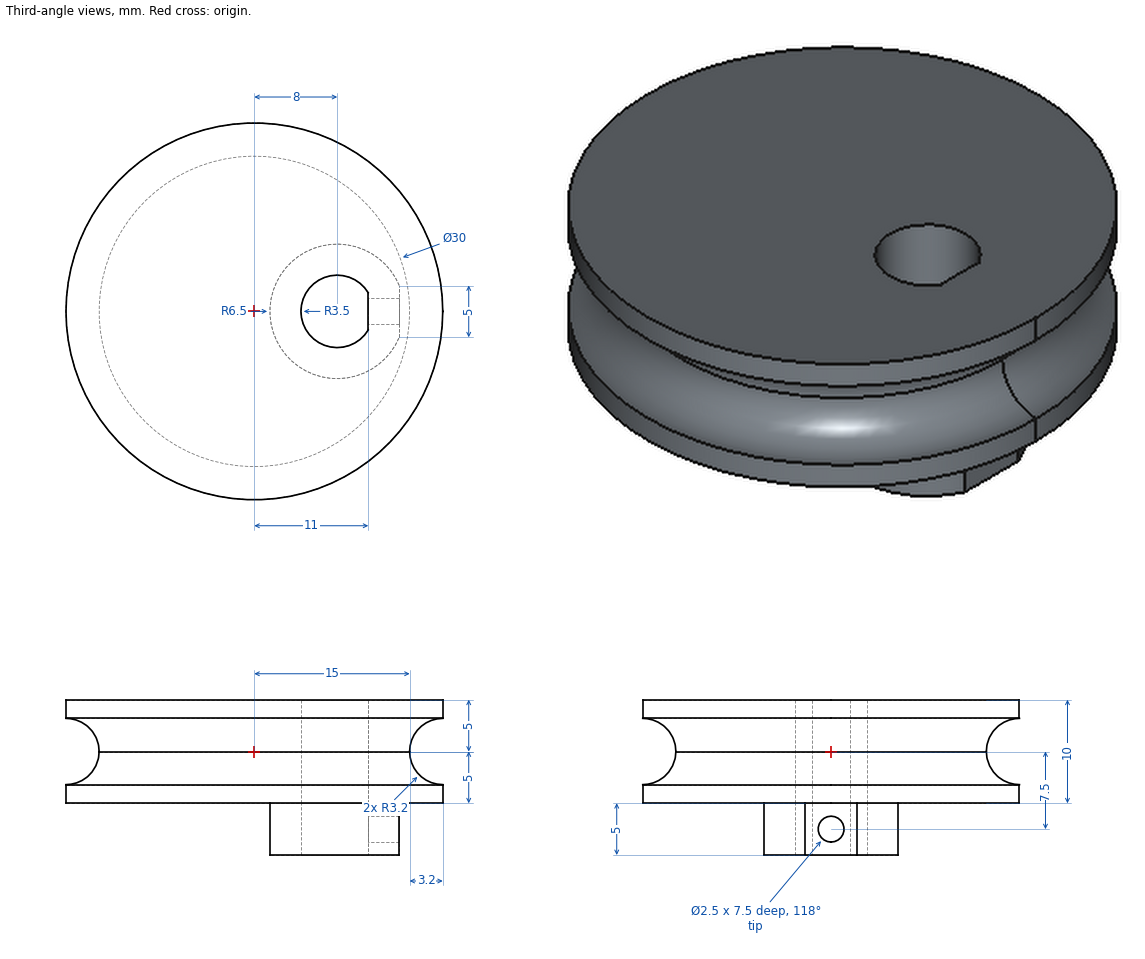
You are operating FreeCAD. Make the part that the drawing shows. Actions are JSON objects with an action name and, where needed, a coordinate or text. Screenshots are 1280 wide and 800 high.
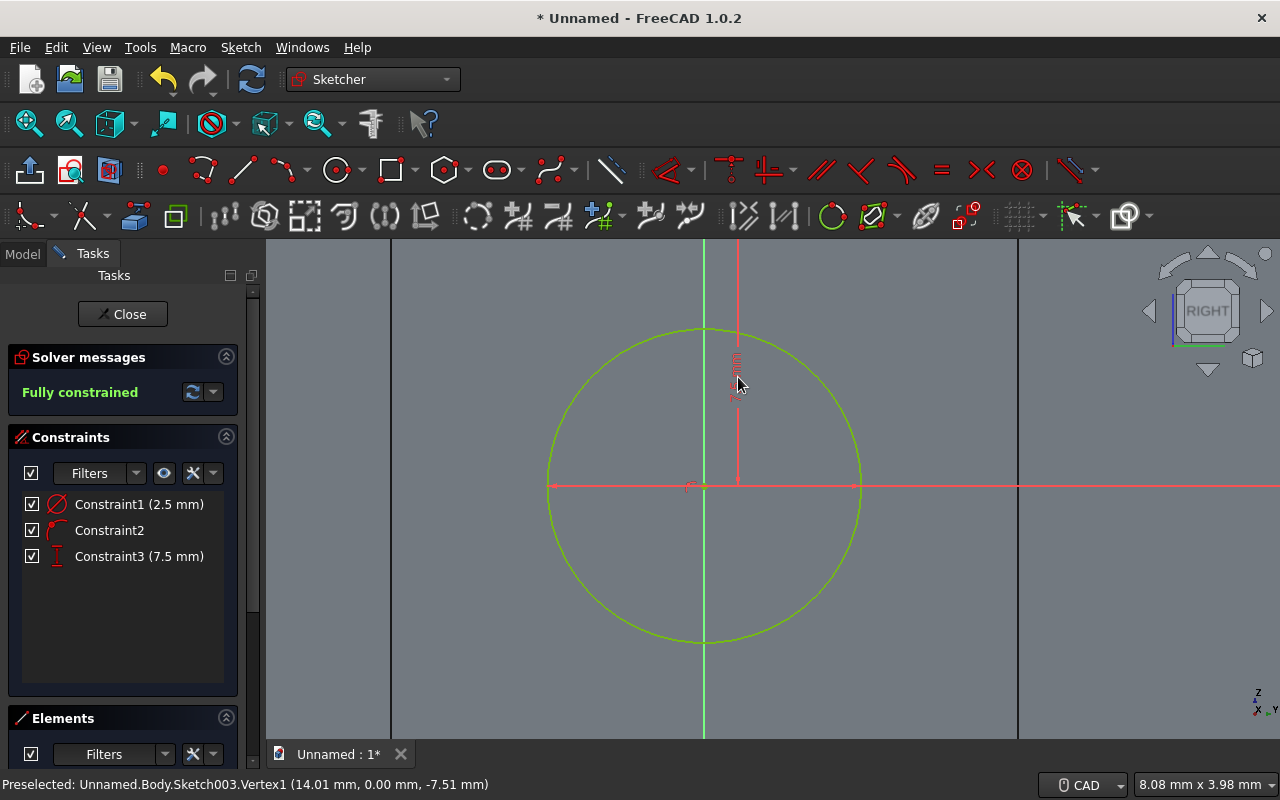
{"action": "left_click", "coordinate": [123, 314]}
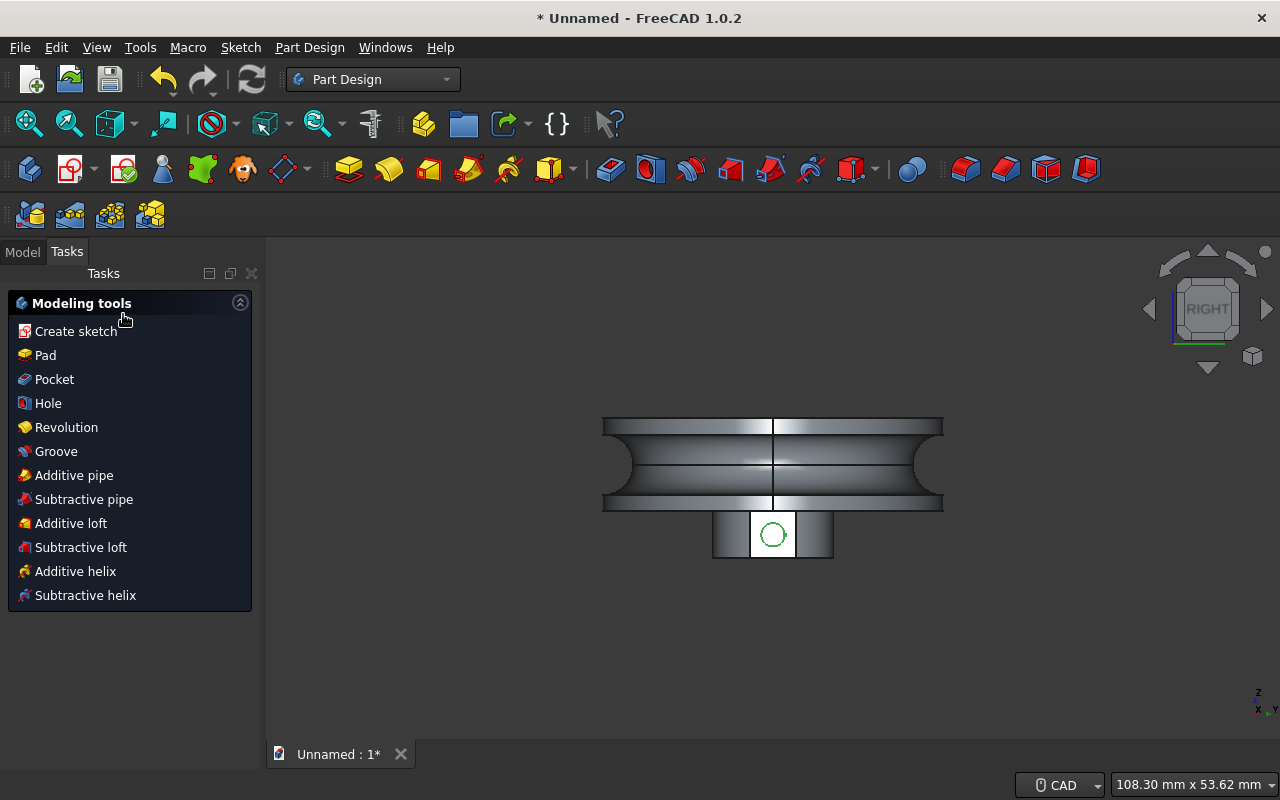
{"action": "left_click", "coordinate": [652, 170]}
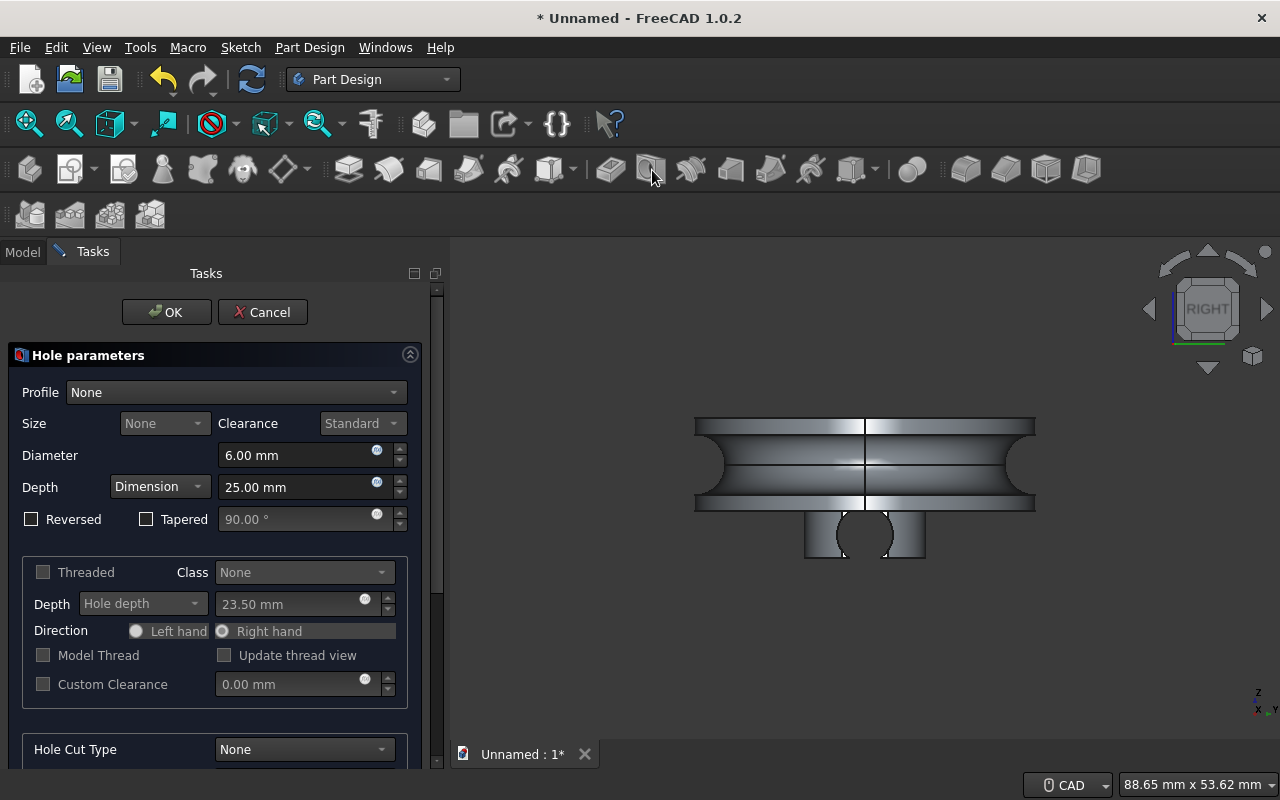
{"action": "triple_click", "coordinate": [305, 455]}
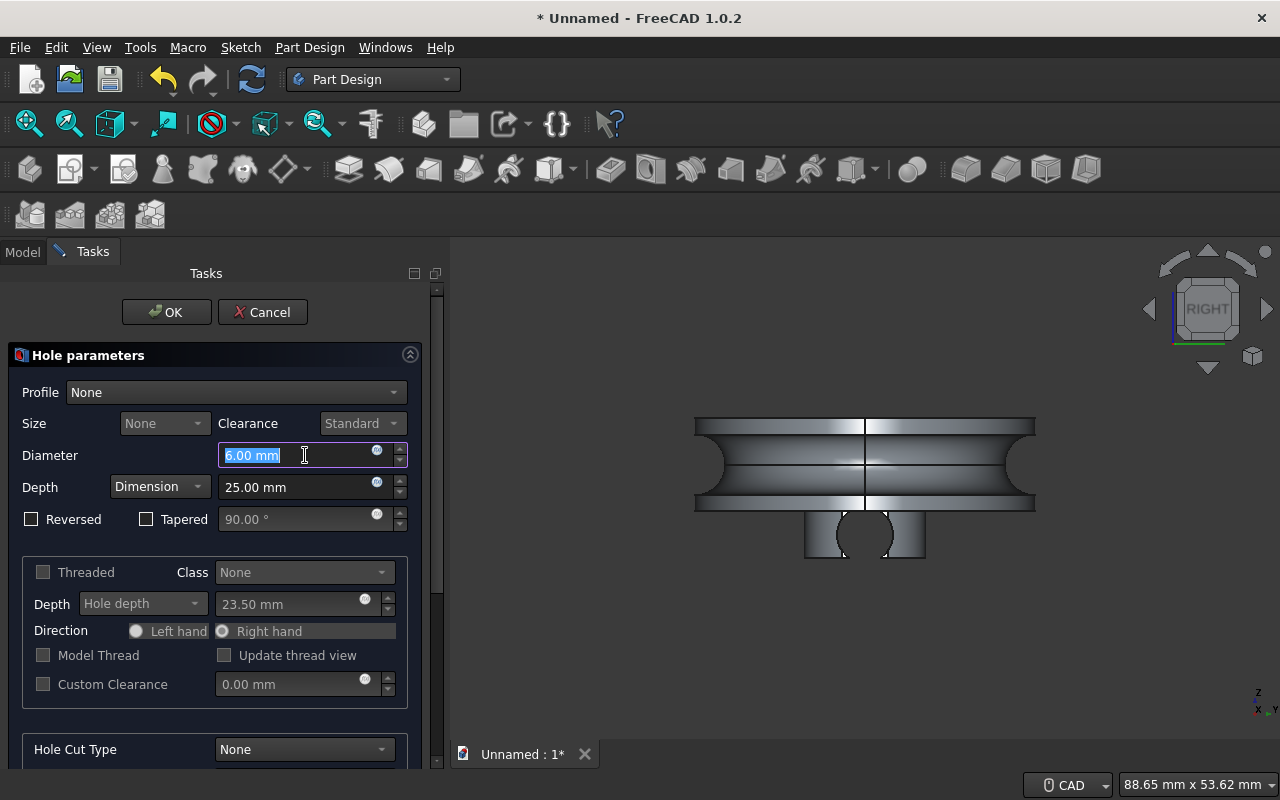
{"action": "type", "text": "2.5"}
{"action": "key", "text": "Tab"}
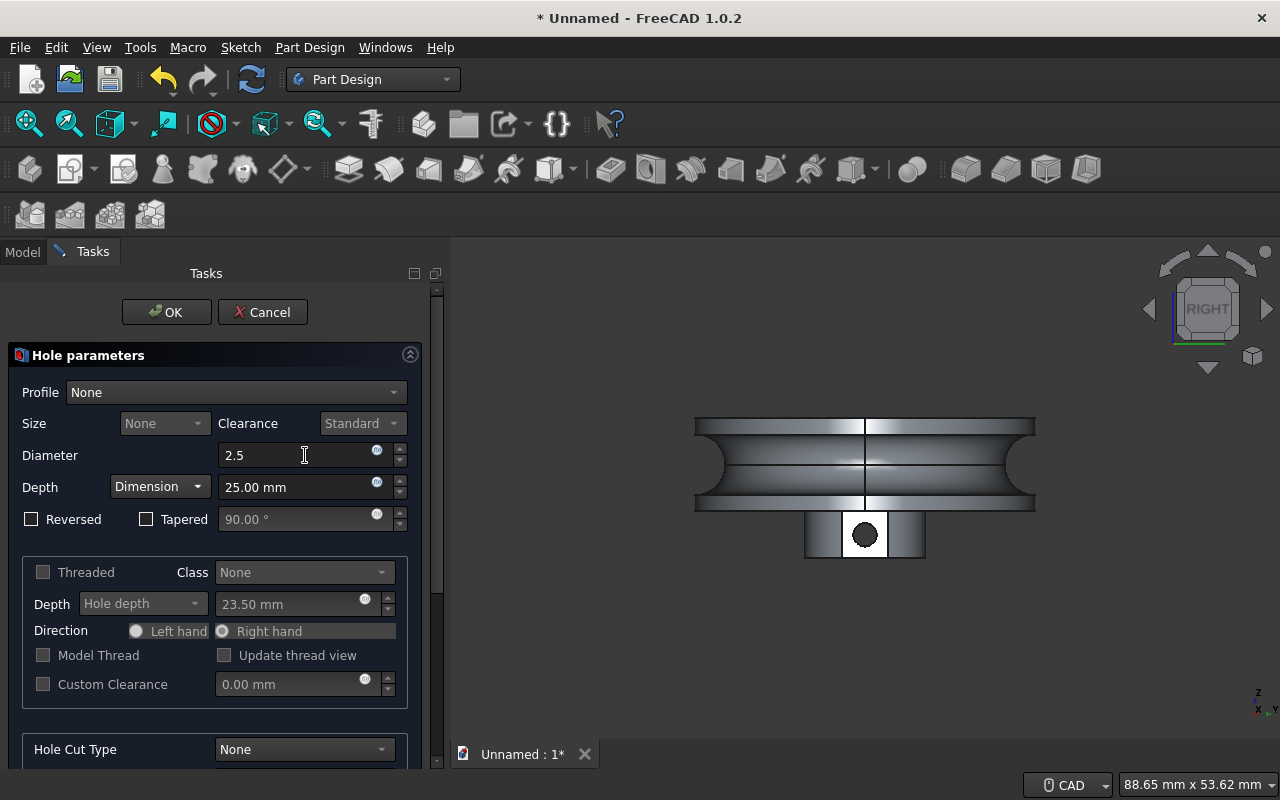
{"action": "triple_click", "coordinate": [305, 487]}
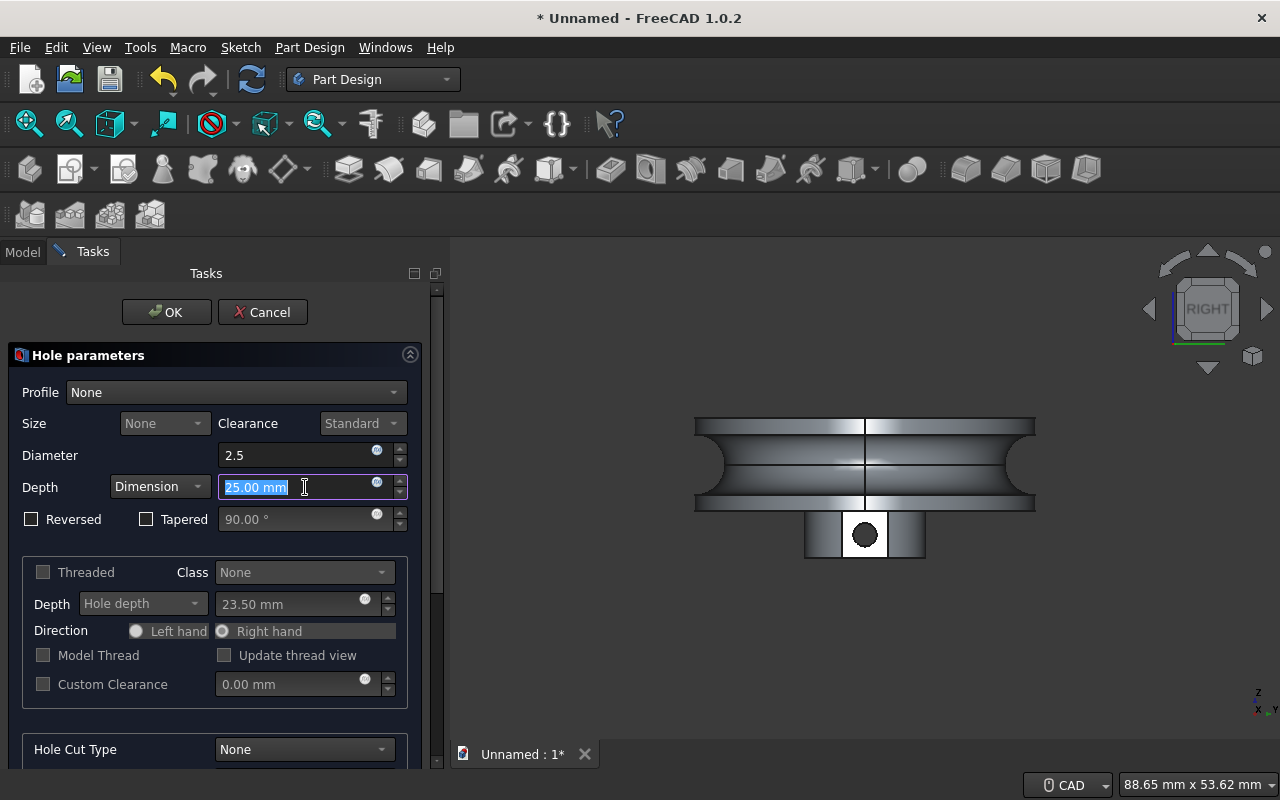
{"action": "type", "text": "7.5"}
{"action": "key", "text": "Tab"}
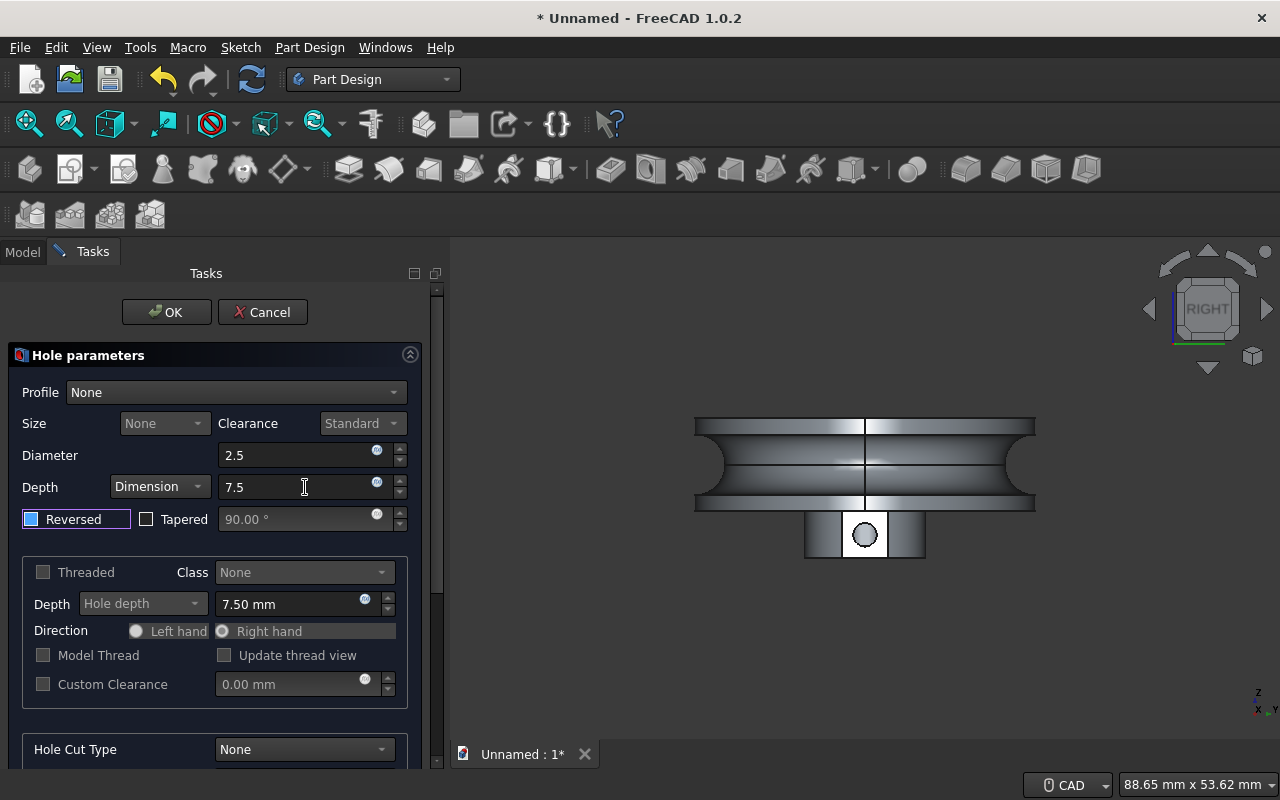
{"action": "left_click", "coordinate": [167, 312]}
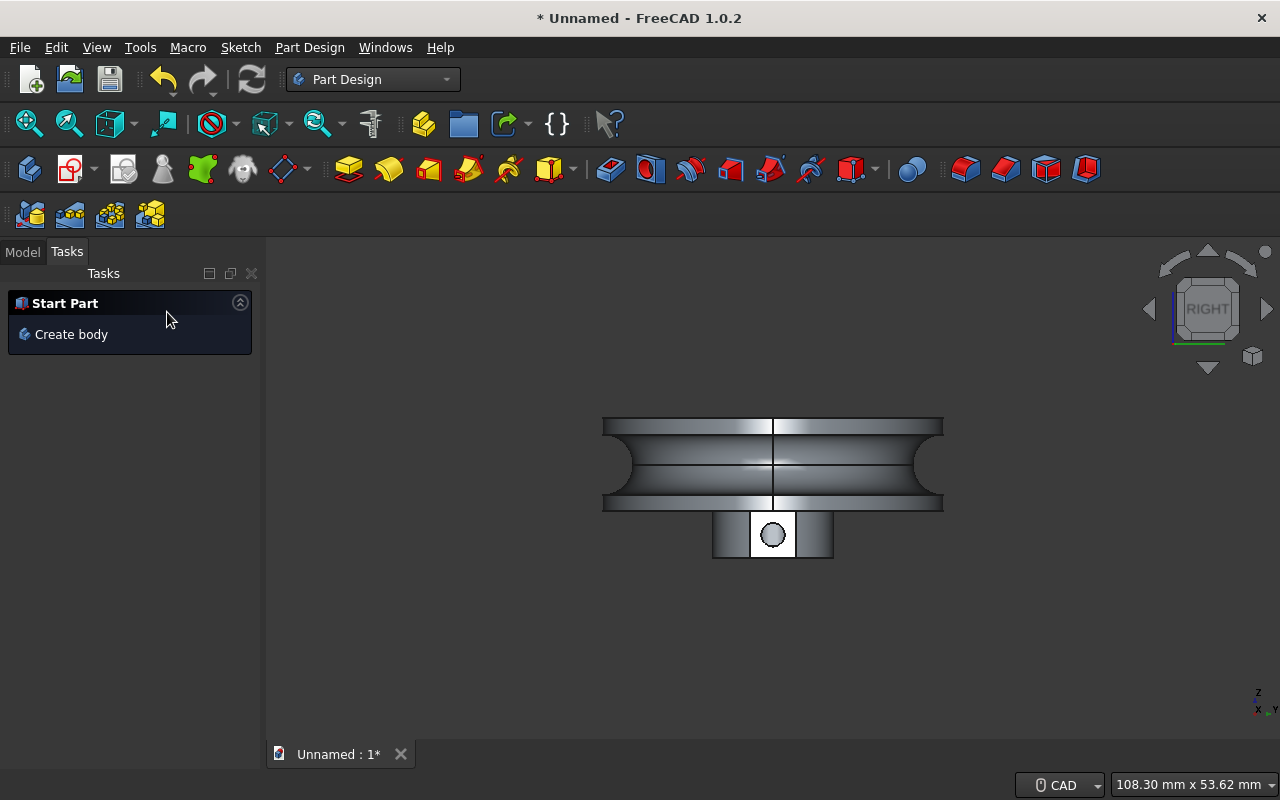
{"action": "key", "text": "0"}